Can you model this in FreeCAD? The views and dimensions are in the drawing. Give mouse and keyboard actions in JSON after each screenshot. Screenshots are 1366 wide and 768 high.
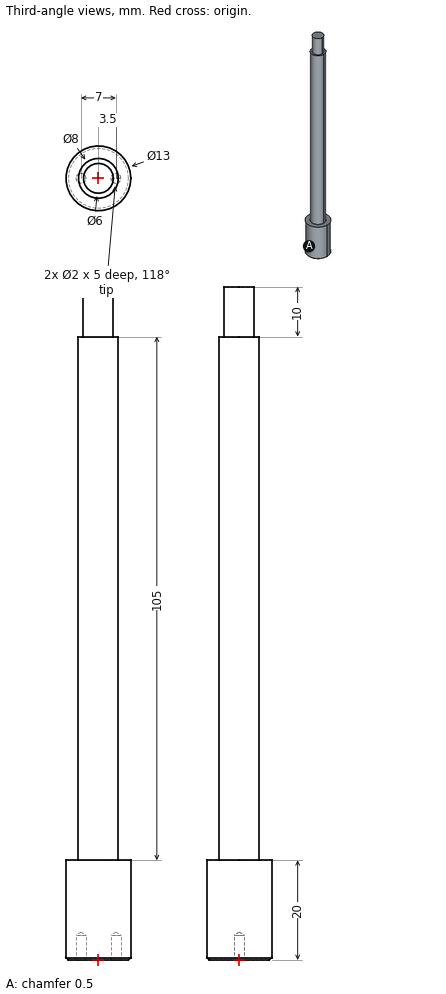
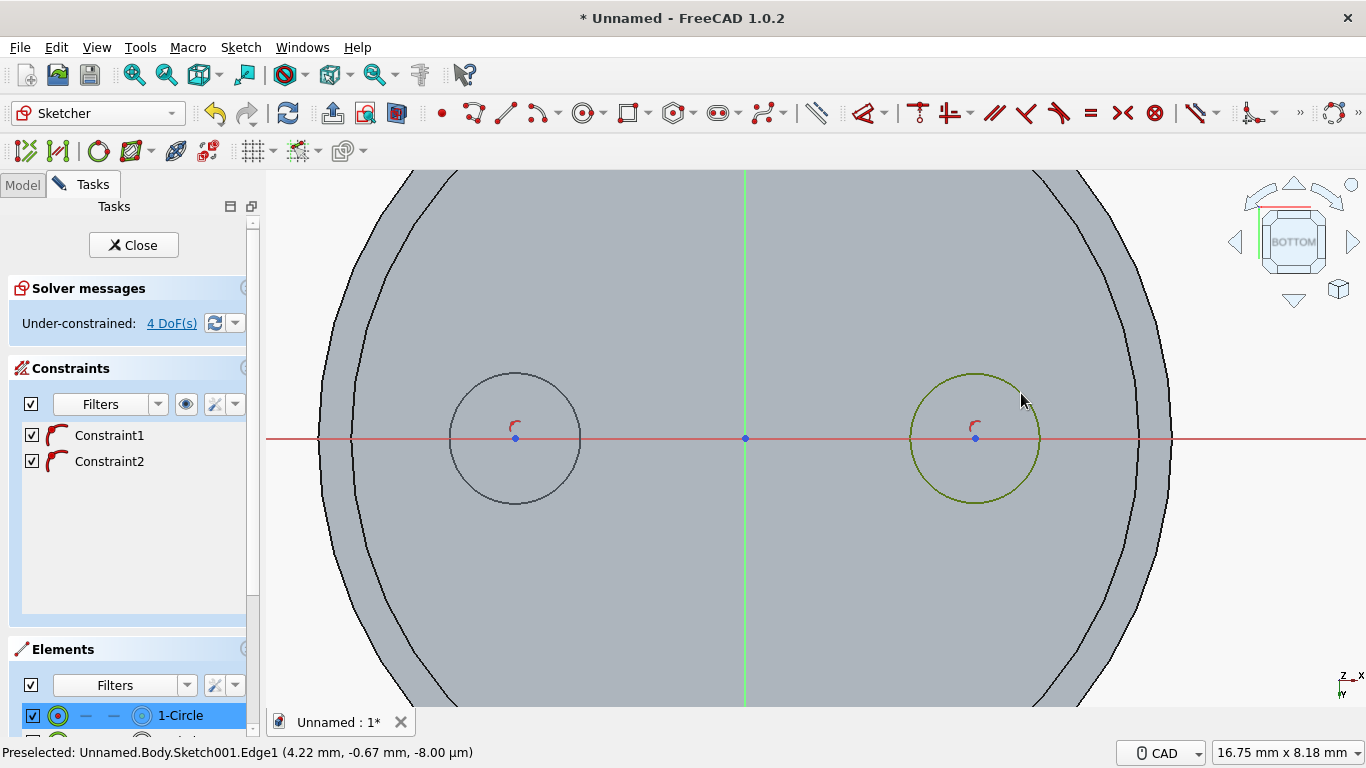
{"action": "left_click", "coordinate": [561, 392]}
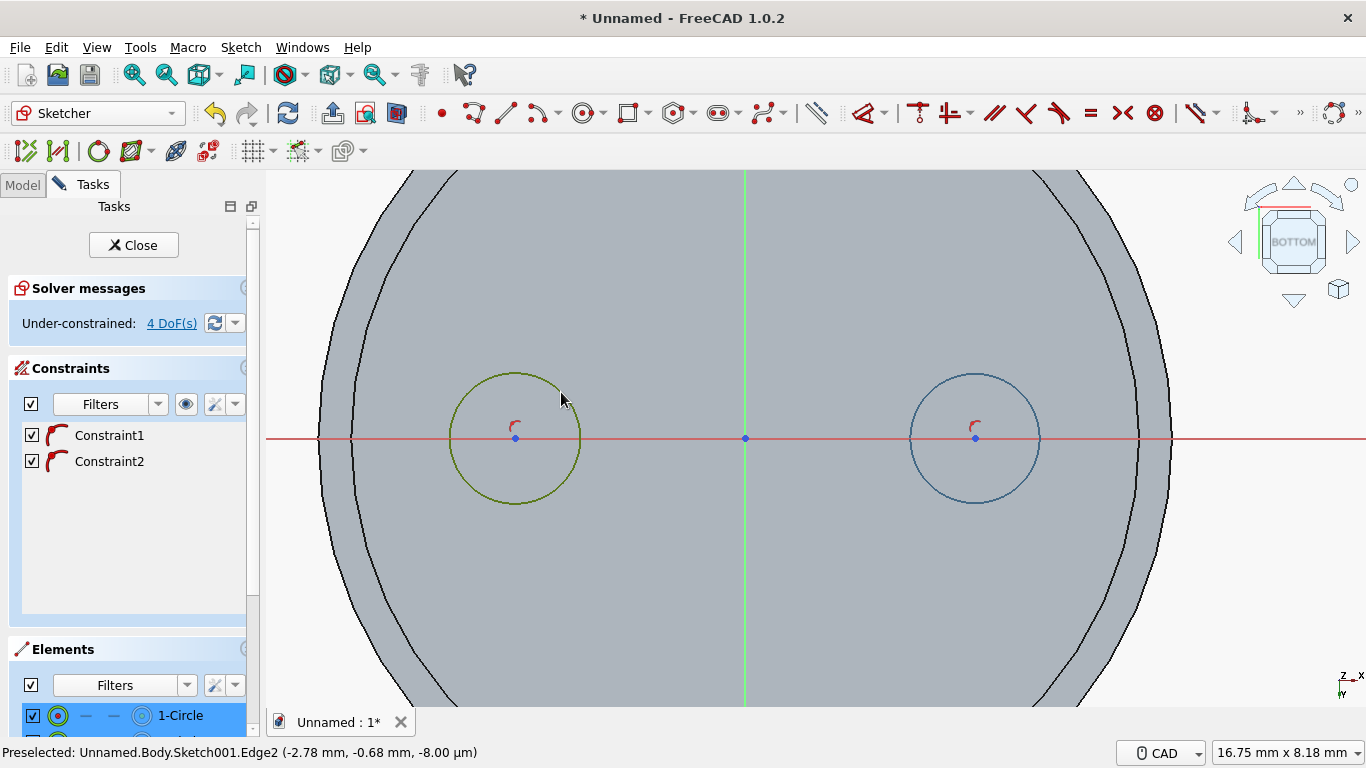
{"action": "key", "text": "e"}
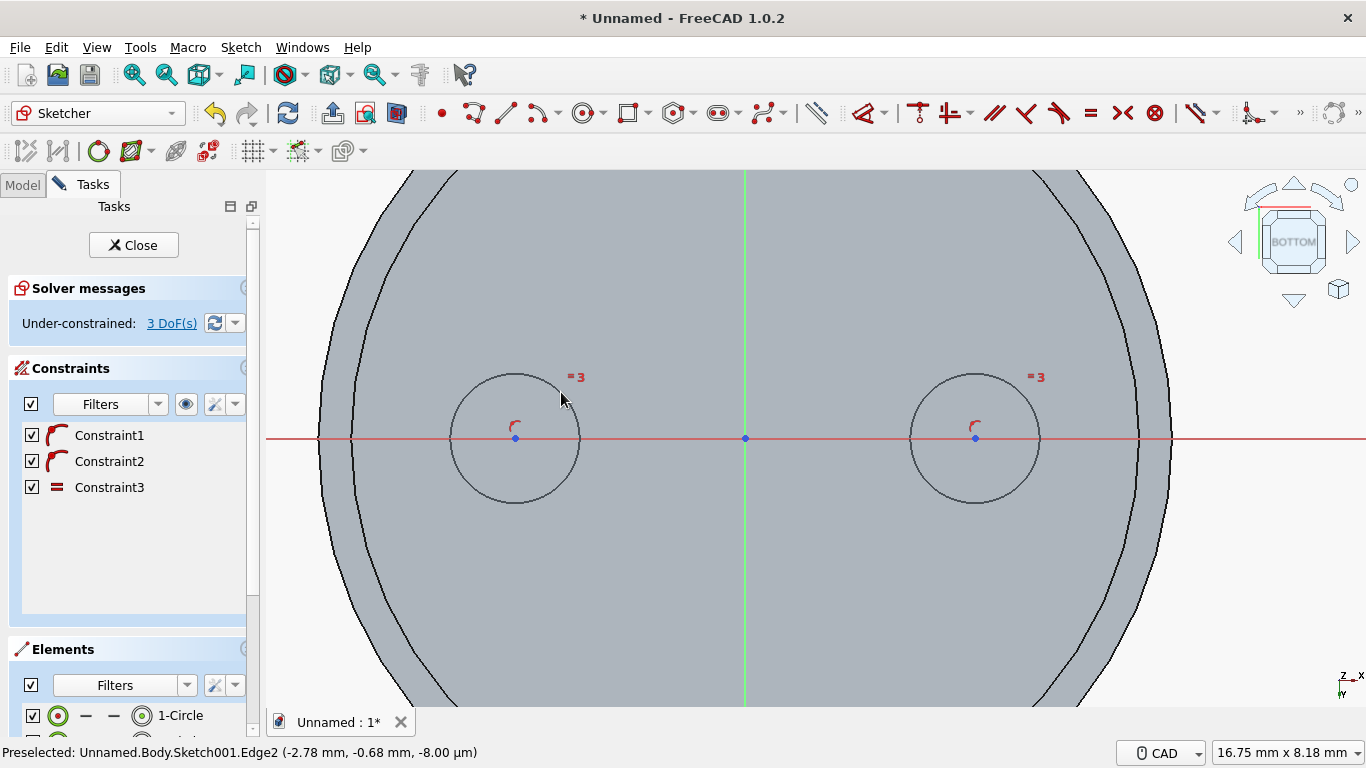
{"action": "left_click", "coordinate": [1021, 393]}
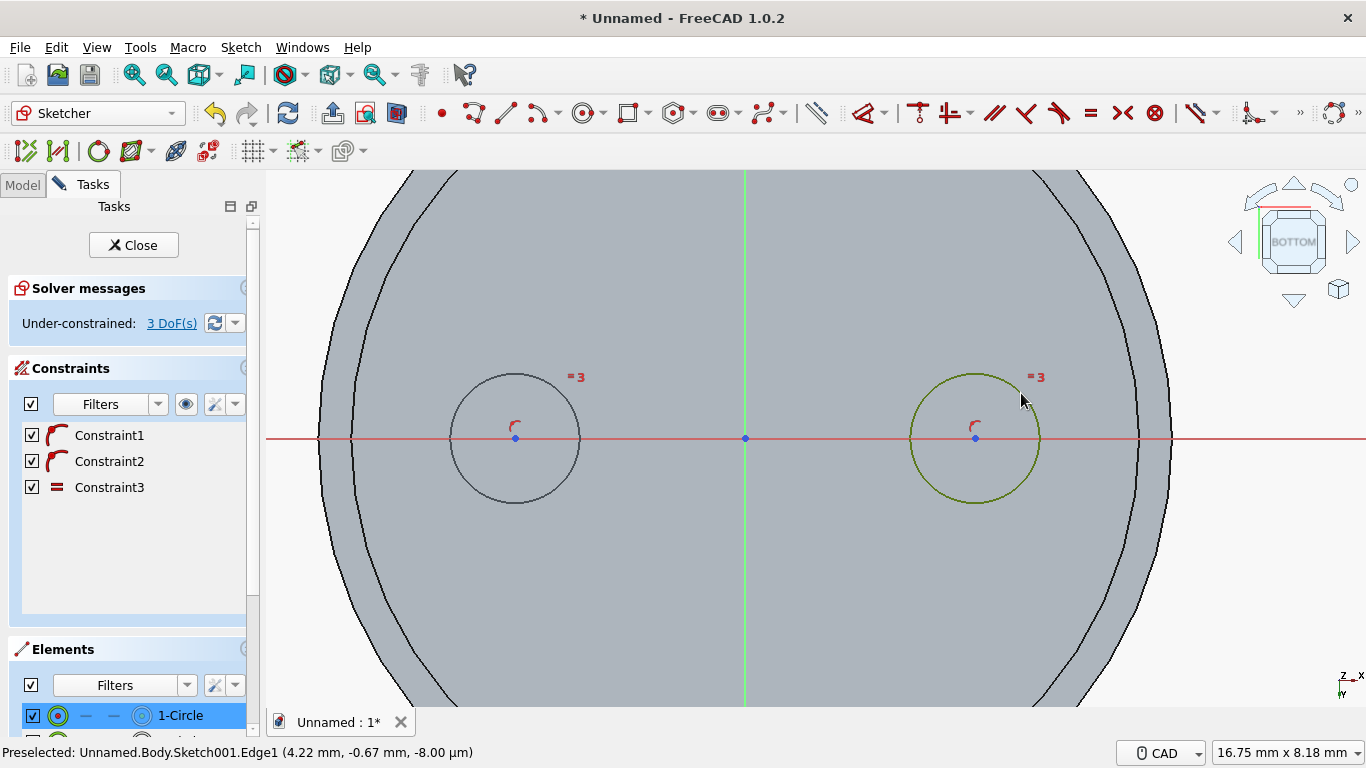
{"action": "key", "text": "k o"}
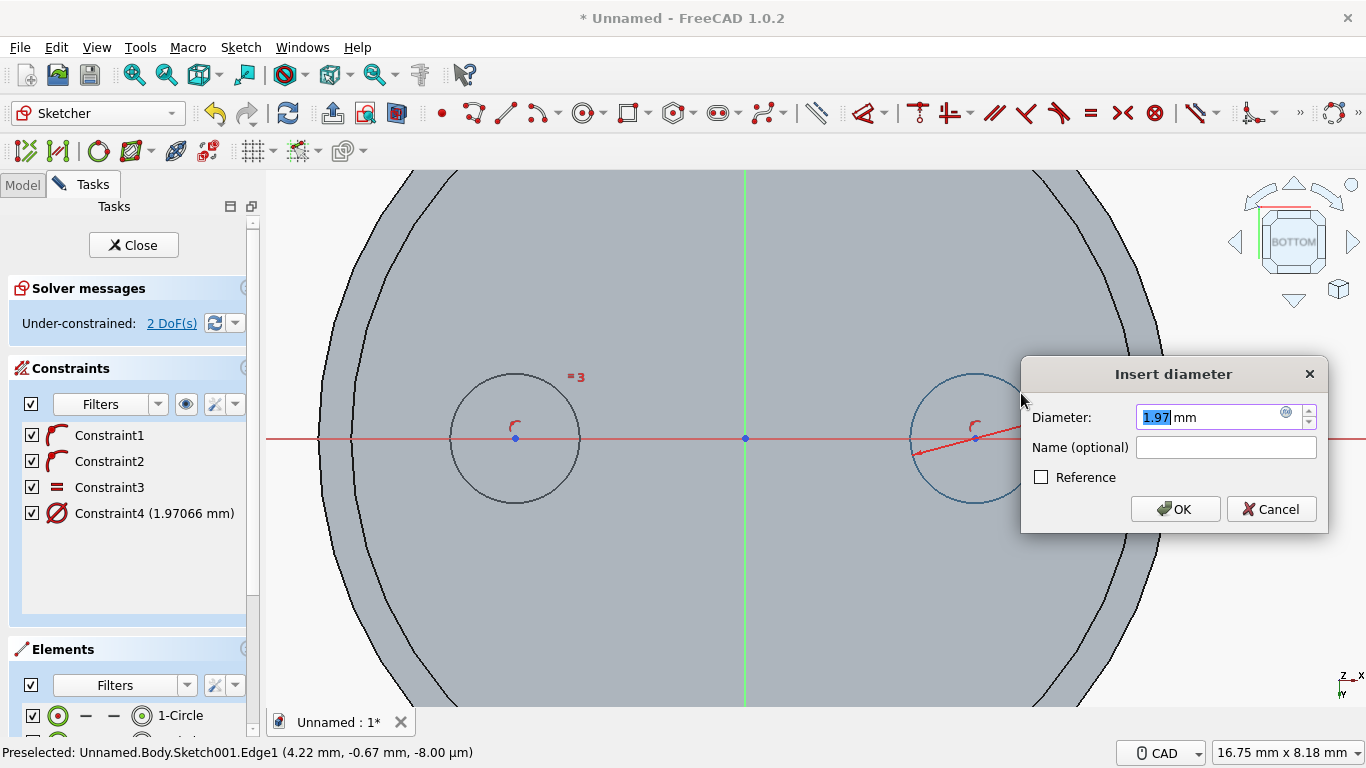
{"action": "type", "text": "2"}
{"action": "key", "text": "Return"}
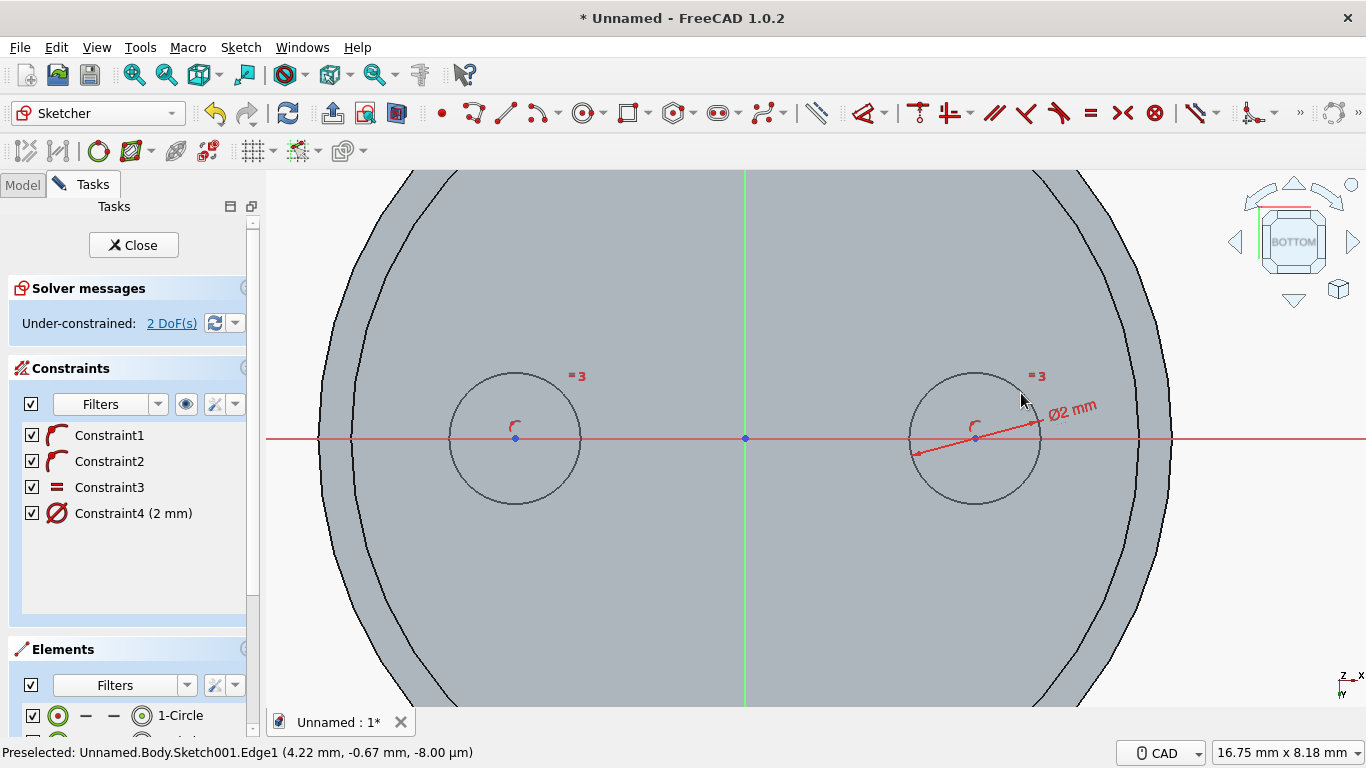
{"action": "left_click", "coordinate": [975, 438]}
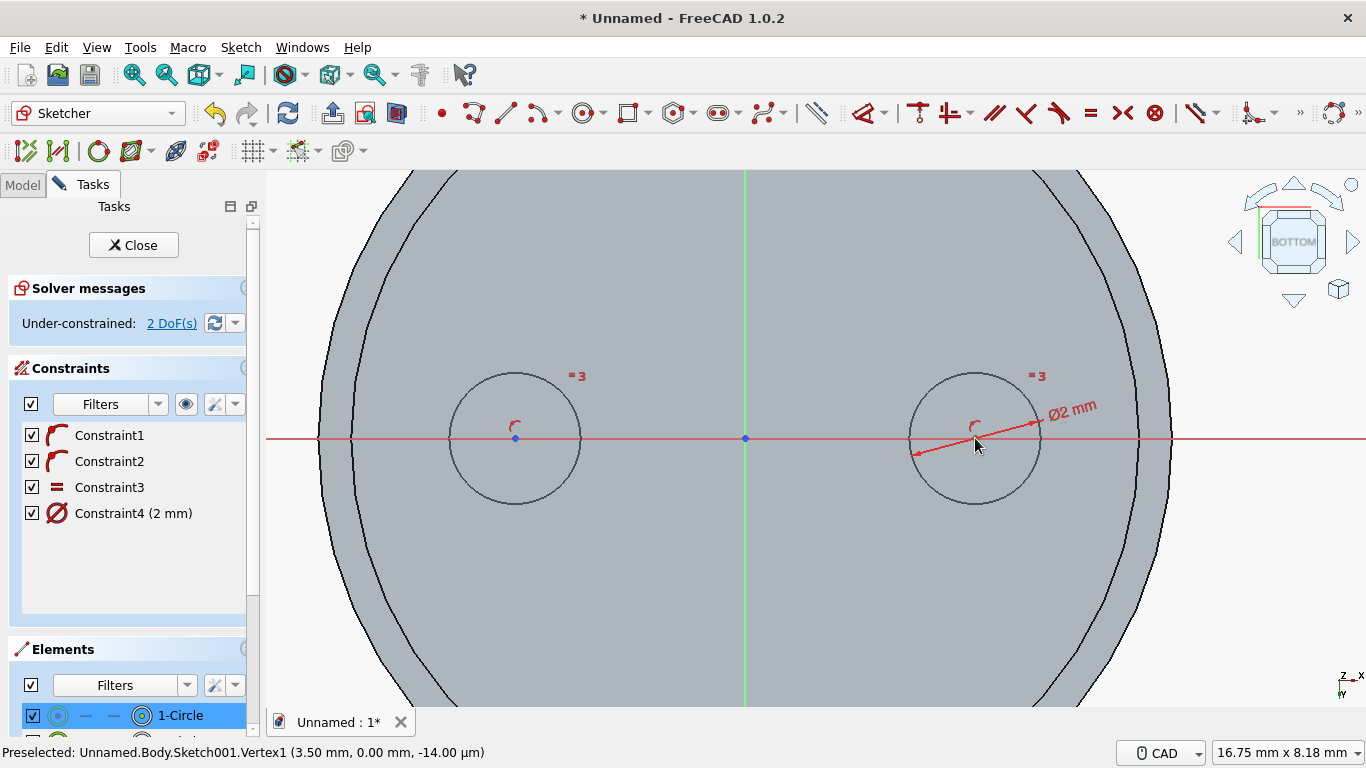
{"action": "left_click", "coordinate": [515, 438]}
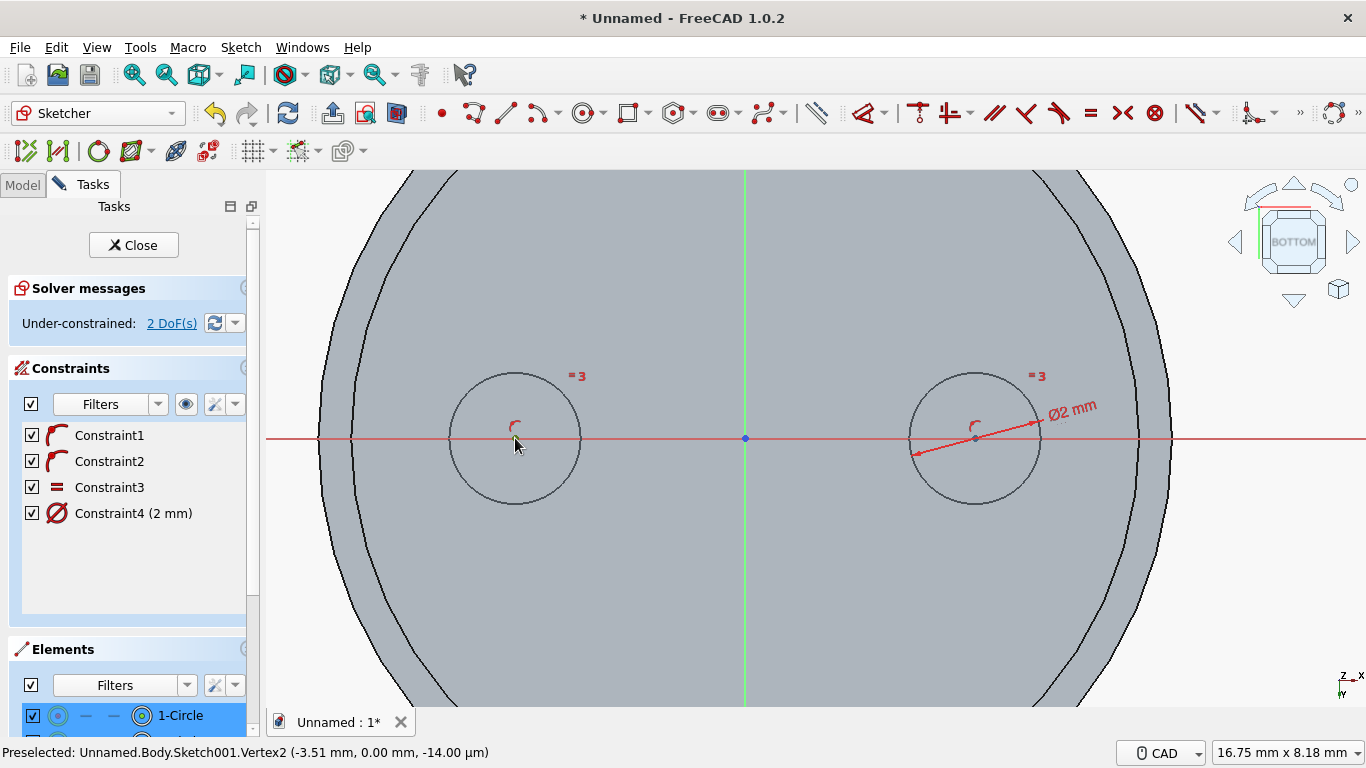
{"action": "left_click", "coordinate": [886, 114]}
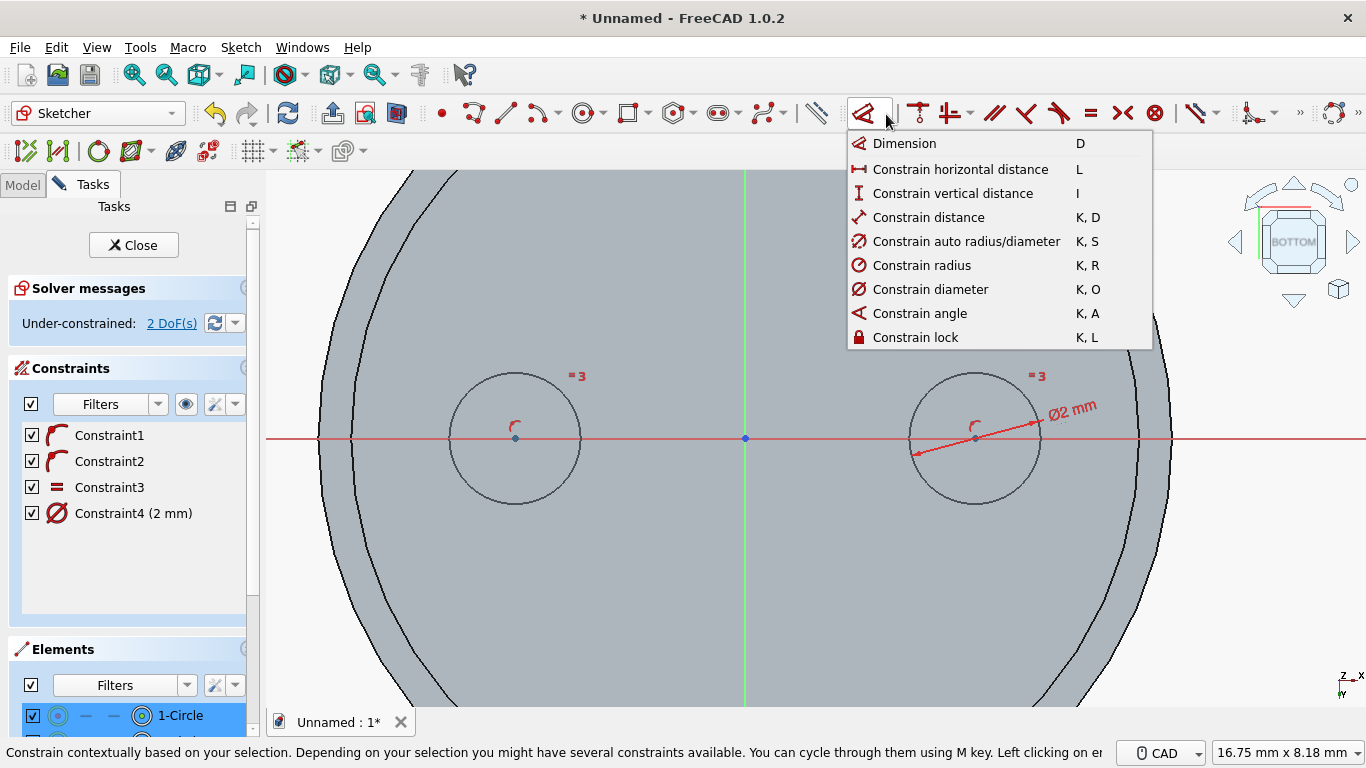
{"action": "left_click", "coordinate": [1000, 169]}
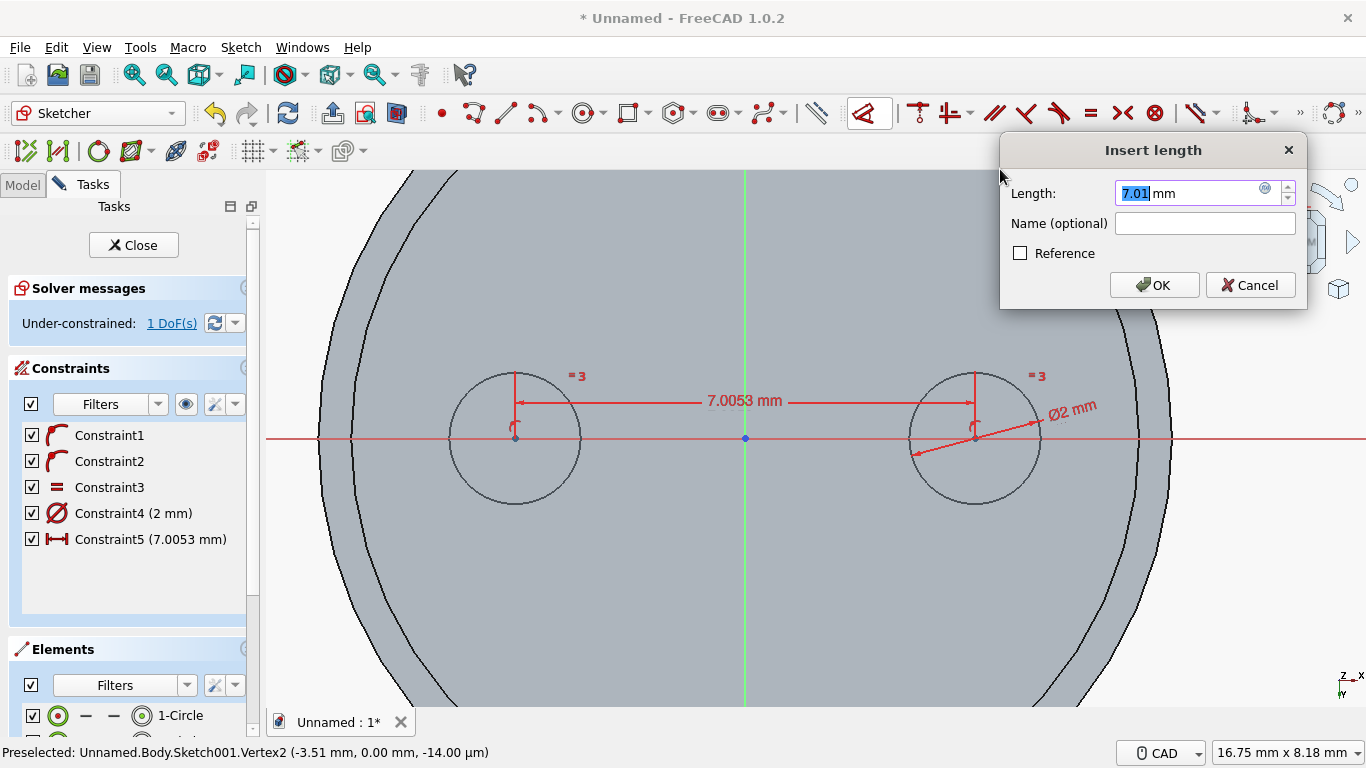
{"action": "type", "text": "7"}
{"action": "key", "text": "Return"}